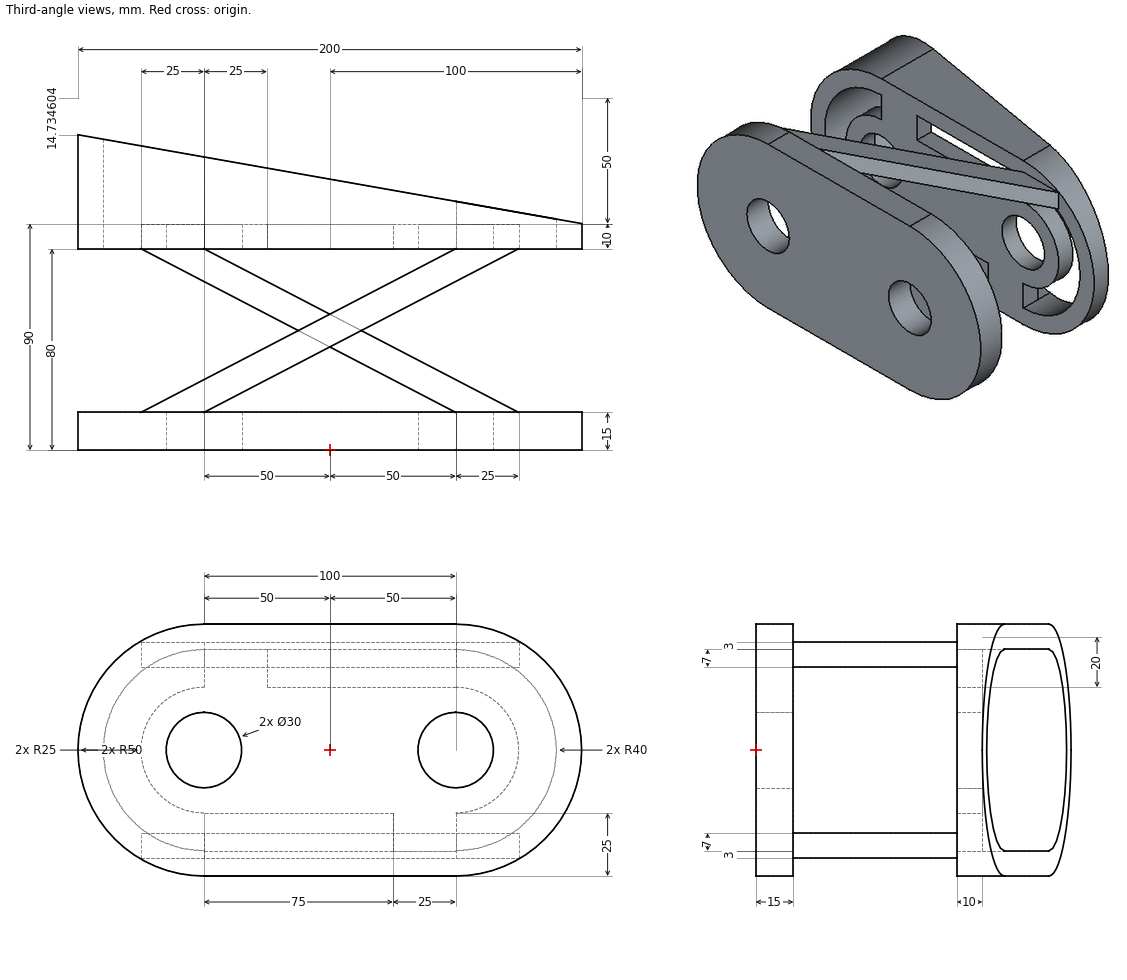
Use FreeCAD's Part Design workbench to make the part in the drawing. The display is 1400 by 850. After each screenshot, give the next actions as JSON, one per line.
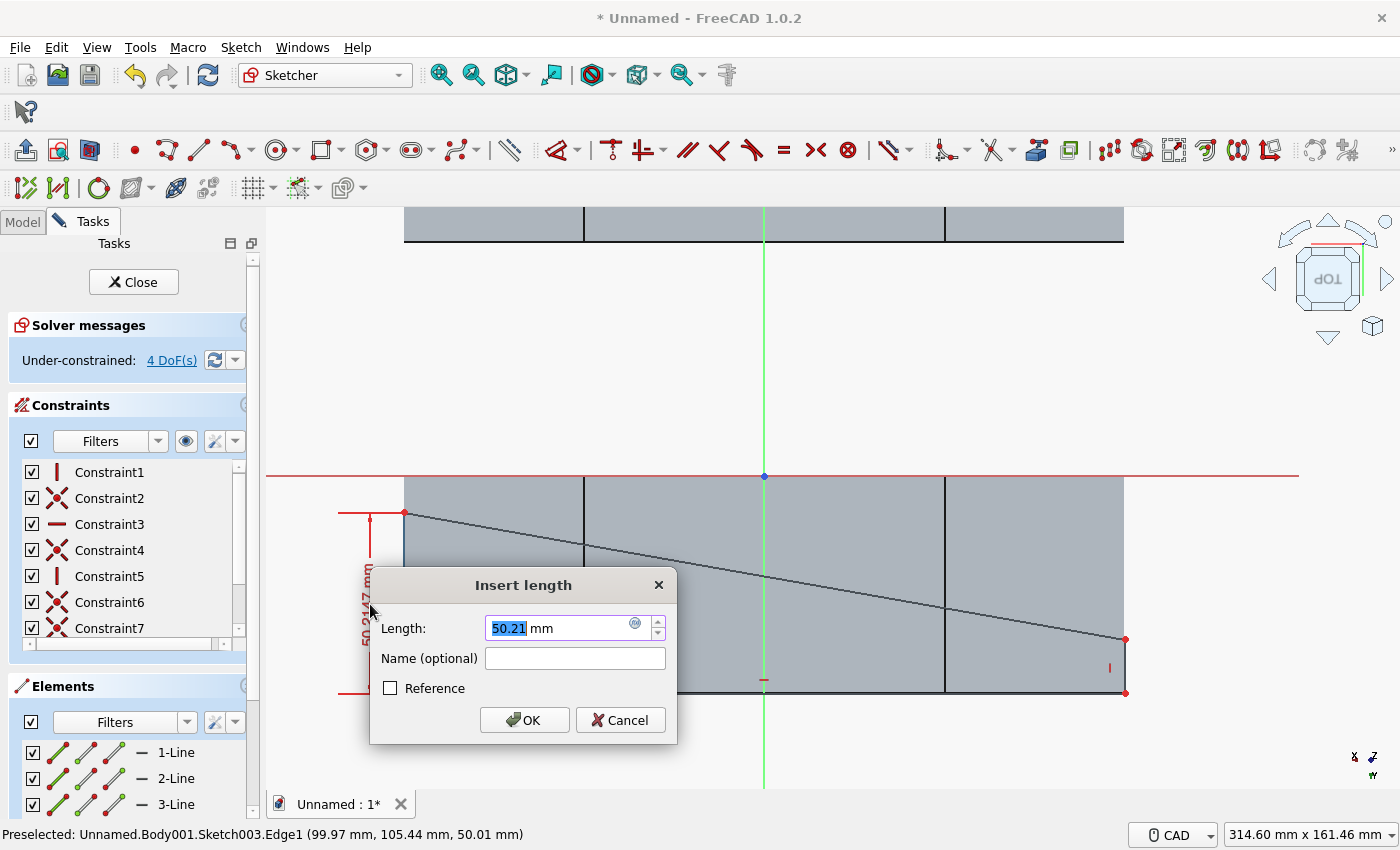
{"action": "type", "text": "50"}
{"action": "key", "text": "Return"}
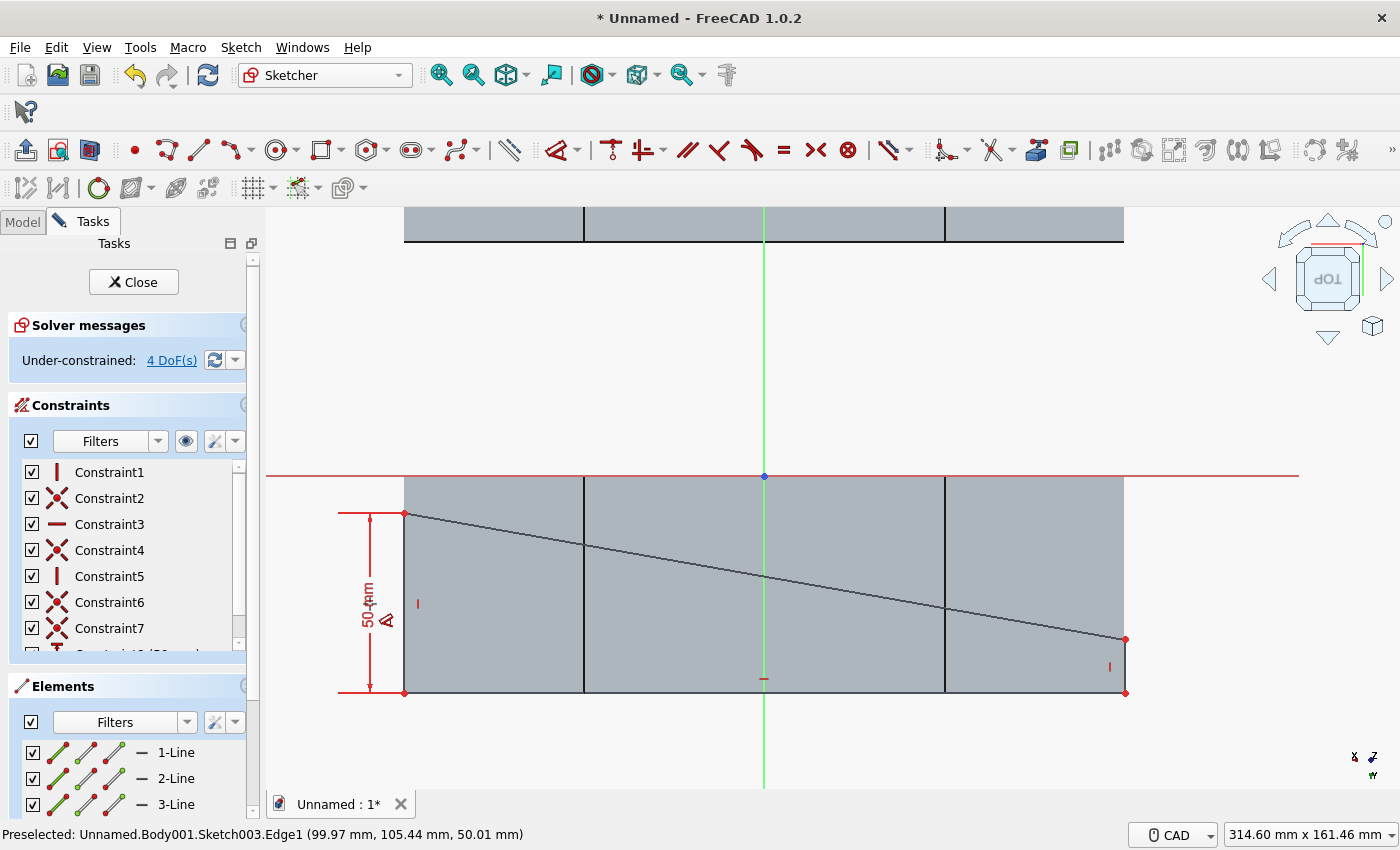
{"action": "left_click", "coordinate": [620, 693]}
{"action": "left_click", "coordinate": [599, 727]}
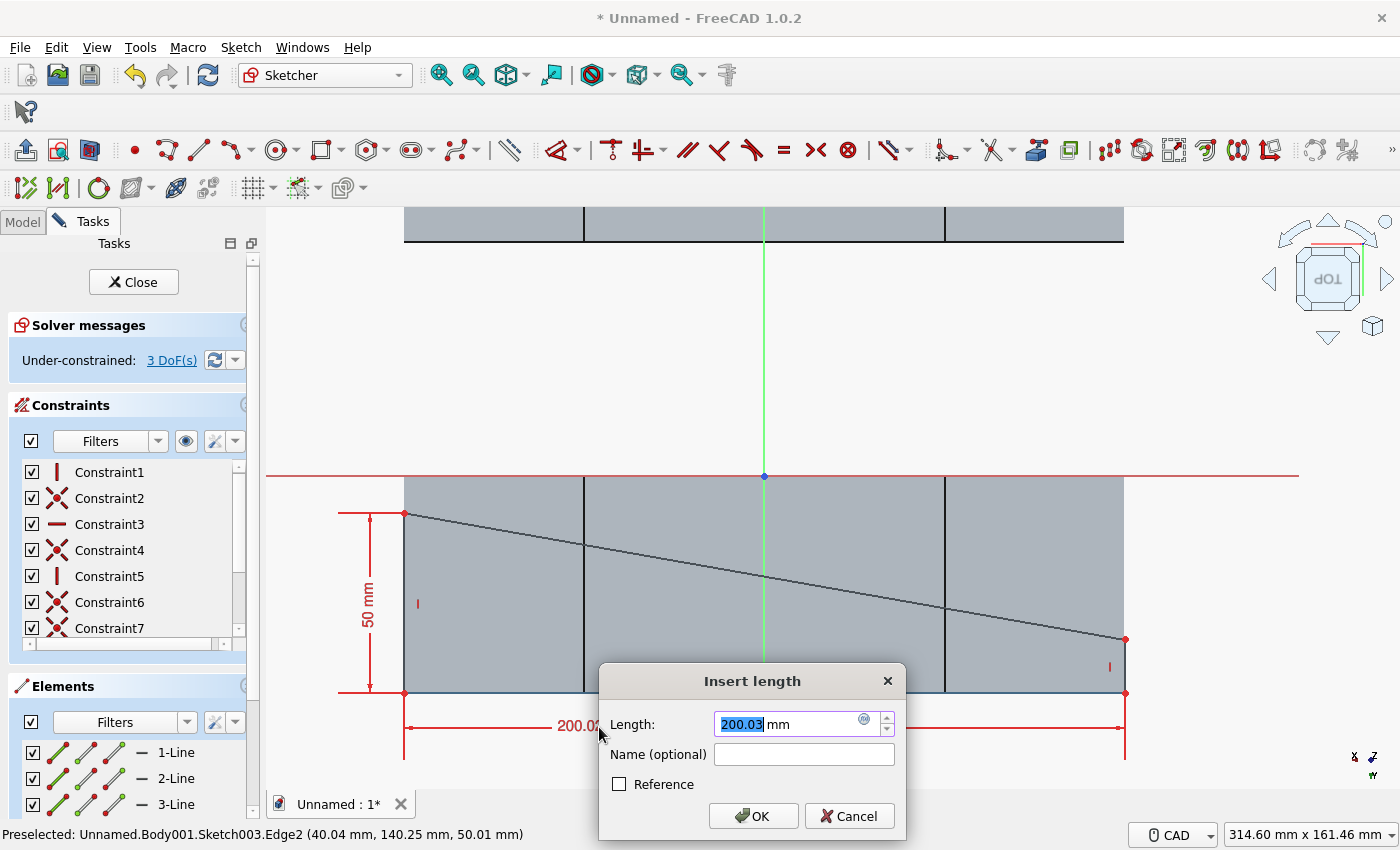
{"action": "type", "text": "200"}
{"action": "key", "text": "Return"}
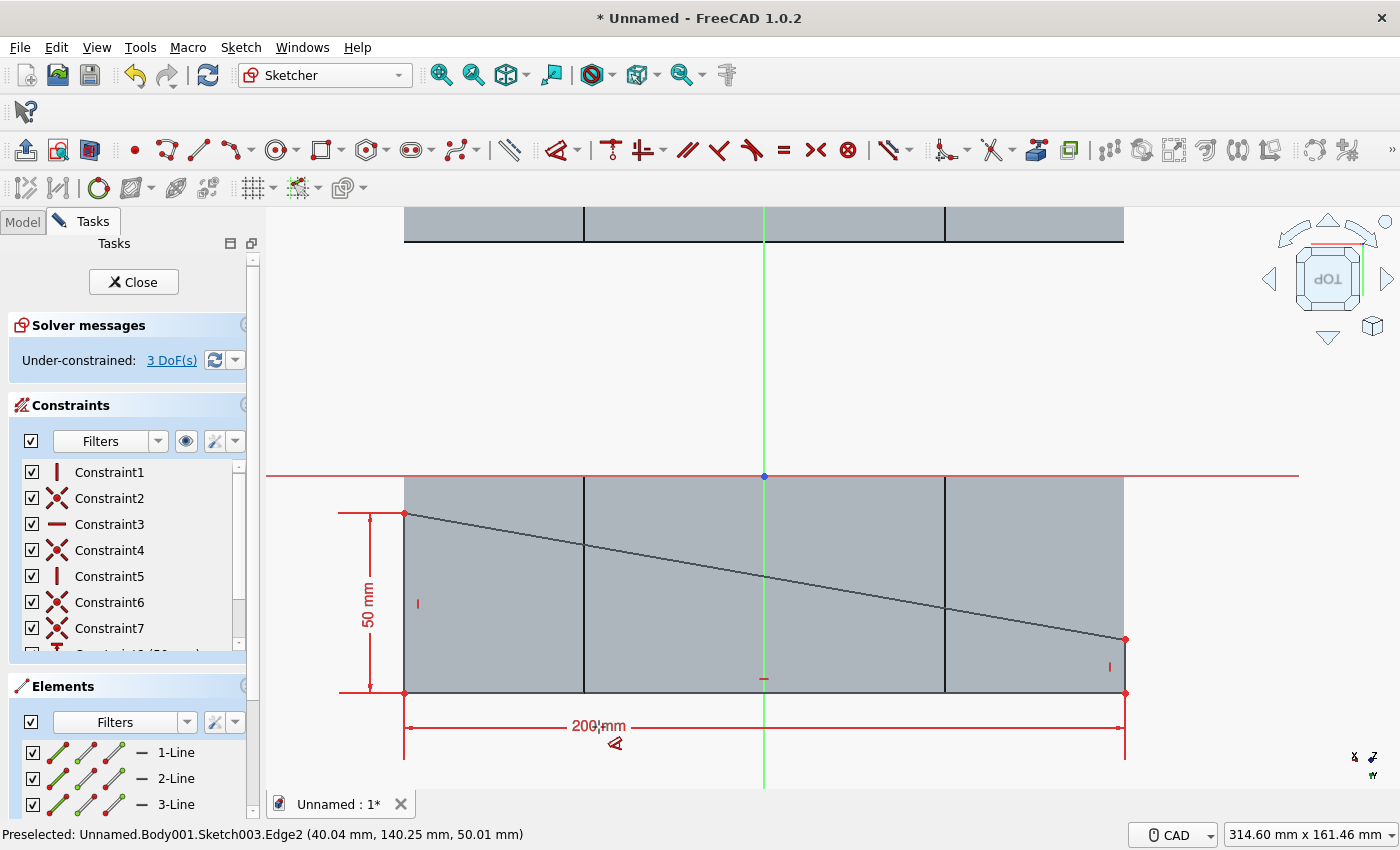
{"action": "left_click", "coordinate": [404, 513]}
{"action": "left_click", "coordinate": [370, 495]}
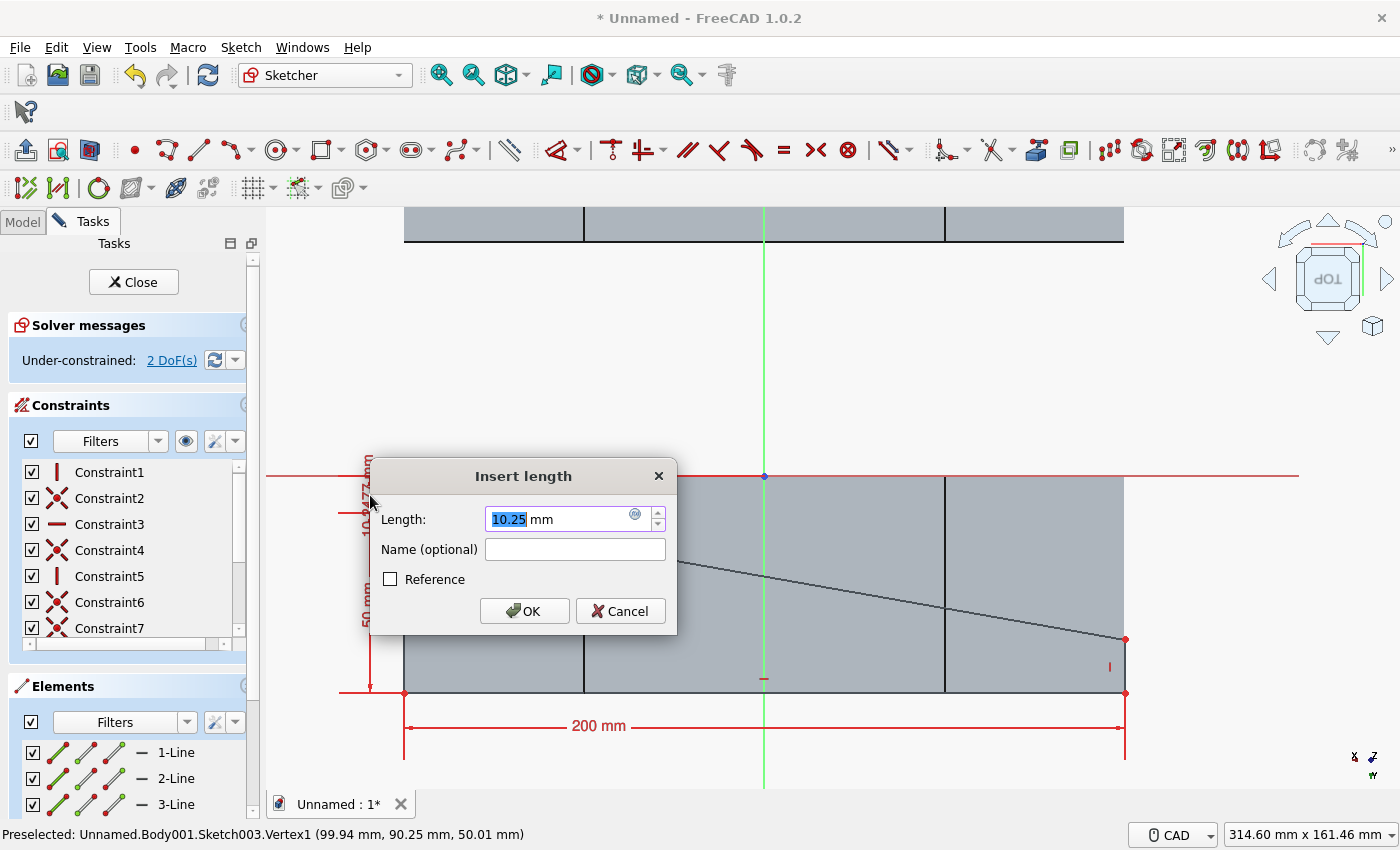
{"action": "type", "text": "10"}
{"action": "key", "text": "Return"}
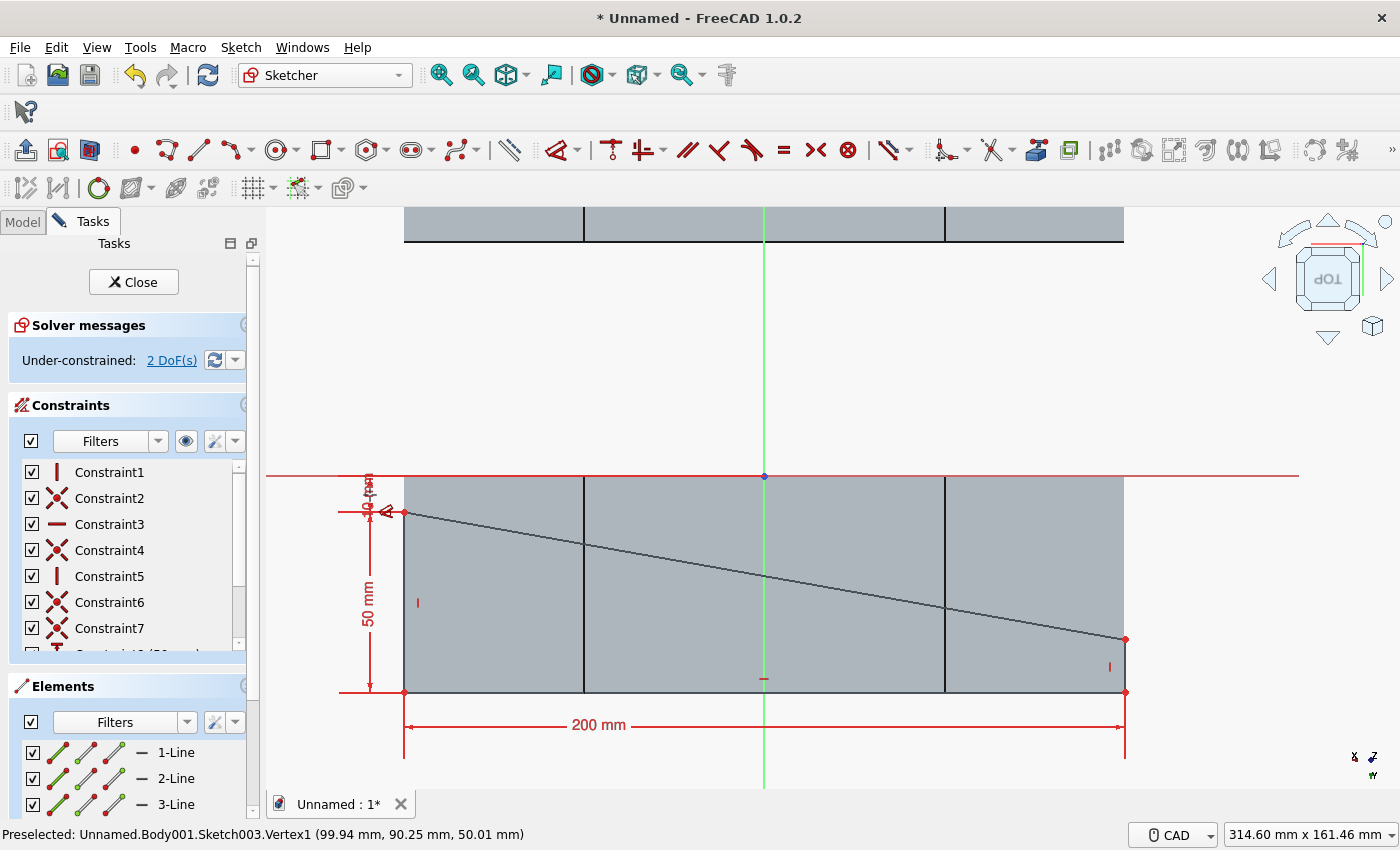
{"action": "left_click", "coordinate": [404, 512]}
{"action": "left_click", "coordinate": [584, 442]}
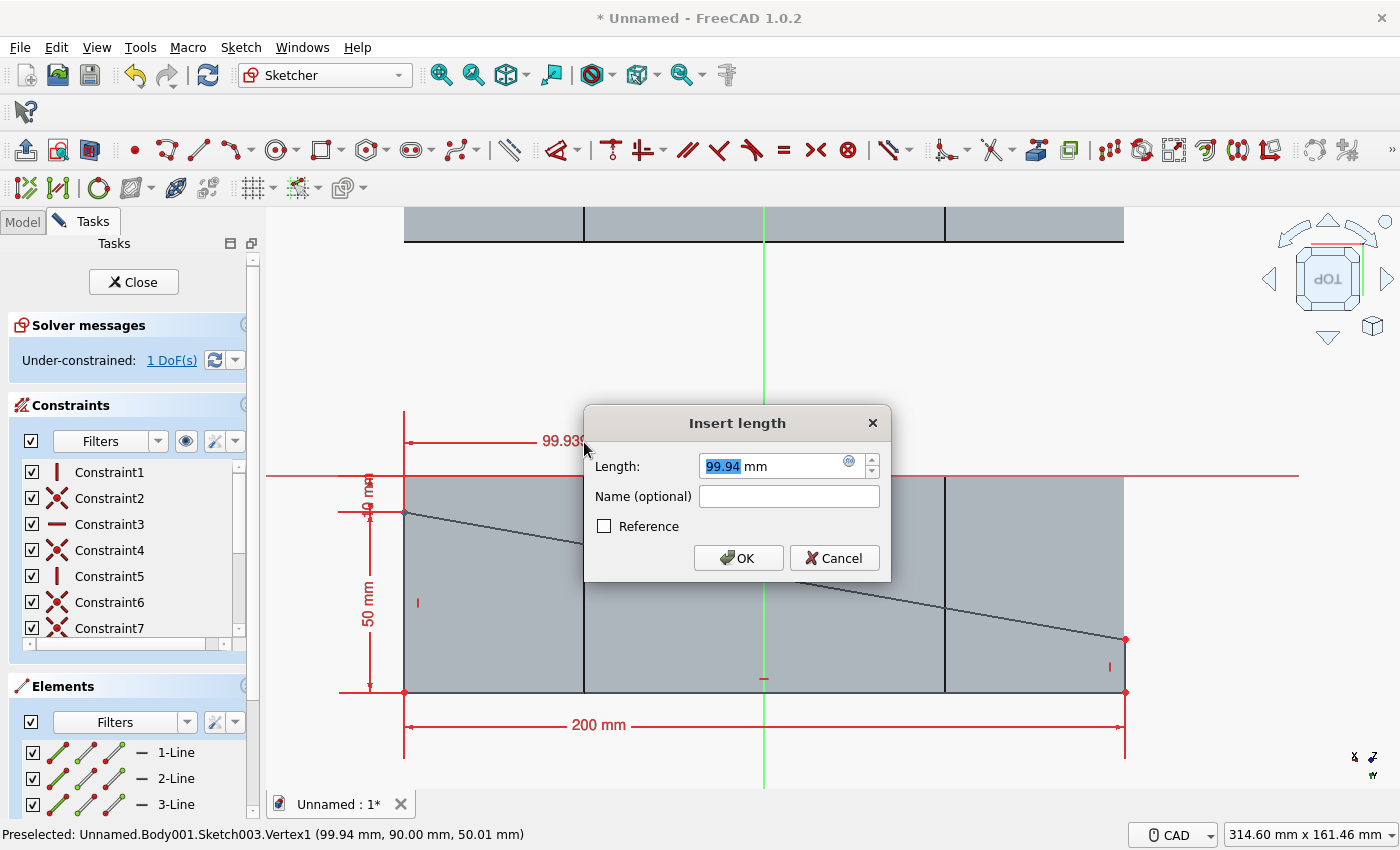
{"action": "type", "text": "100"}
{"action": "key", "text": "Return"}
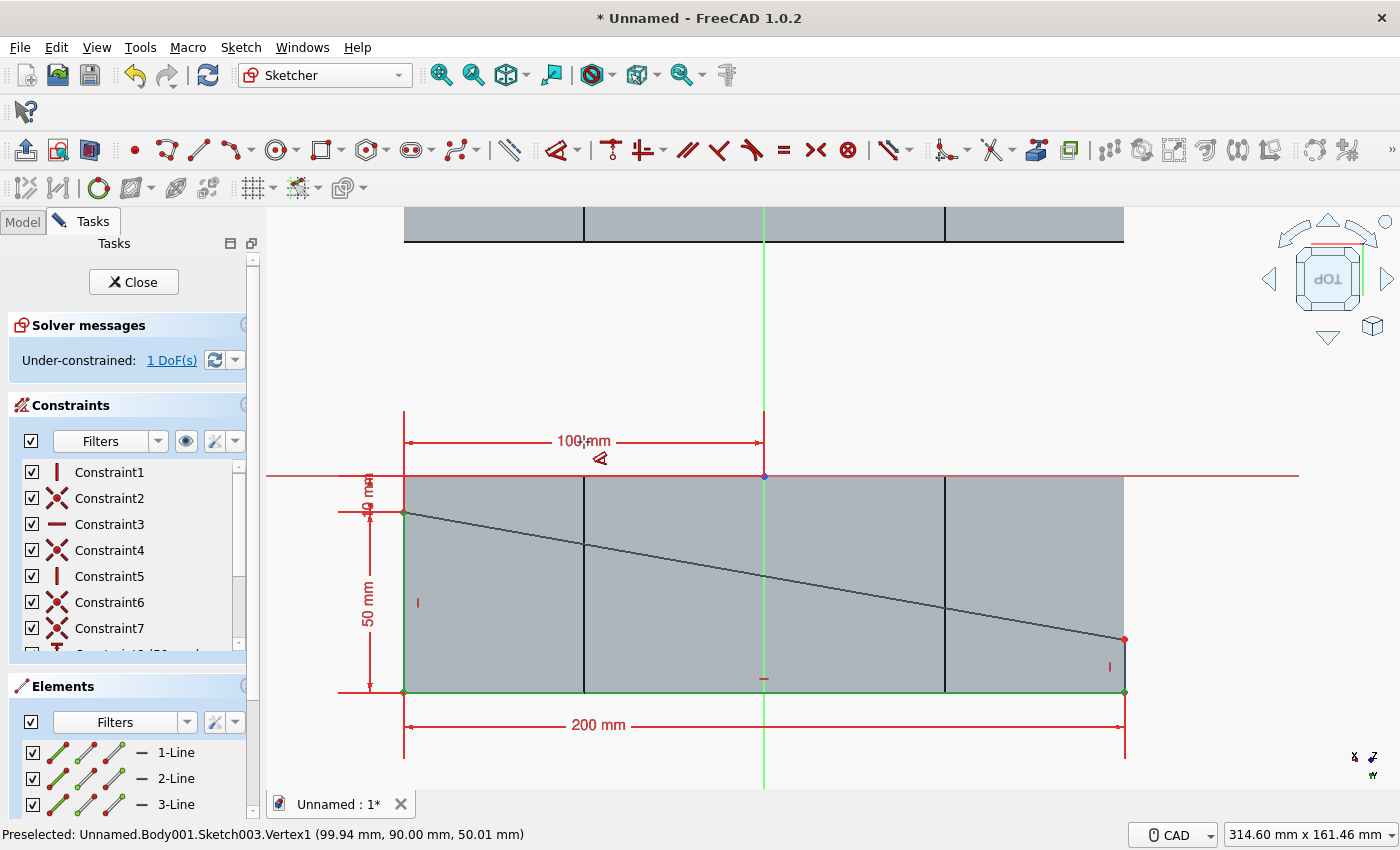
{"action": "left_click", "coordinate": [1125, 677]}
{"action": "left_click", "coordinate": [1159, 666]}